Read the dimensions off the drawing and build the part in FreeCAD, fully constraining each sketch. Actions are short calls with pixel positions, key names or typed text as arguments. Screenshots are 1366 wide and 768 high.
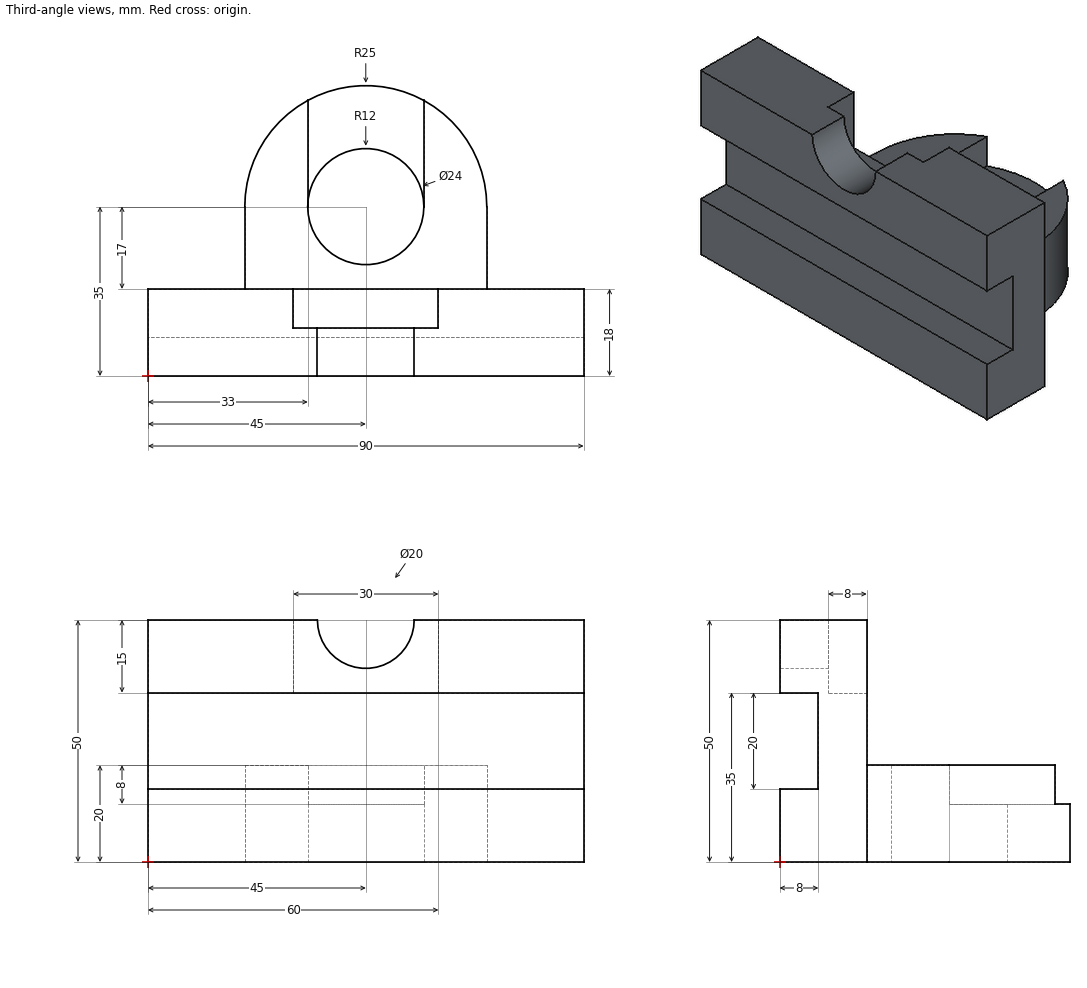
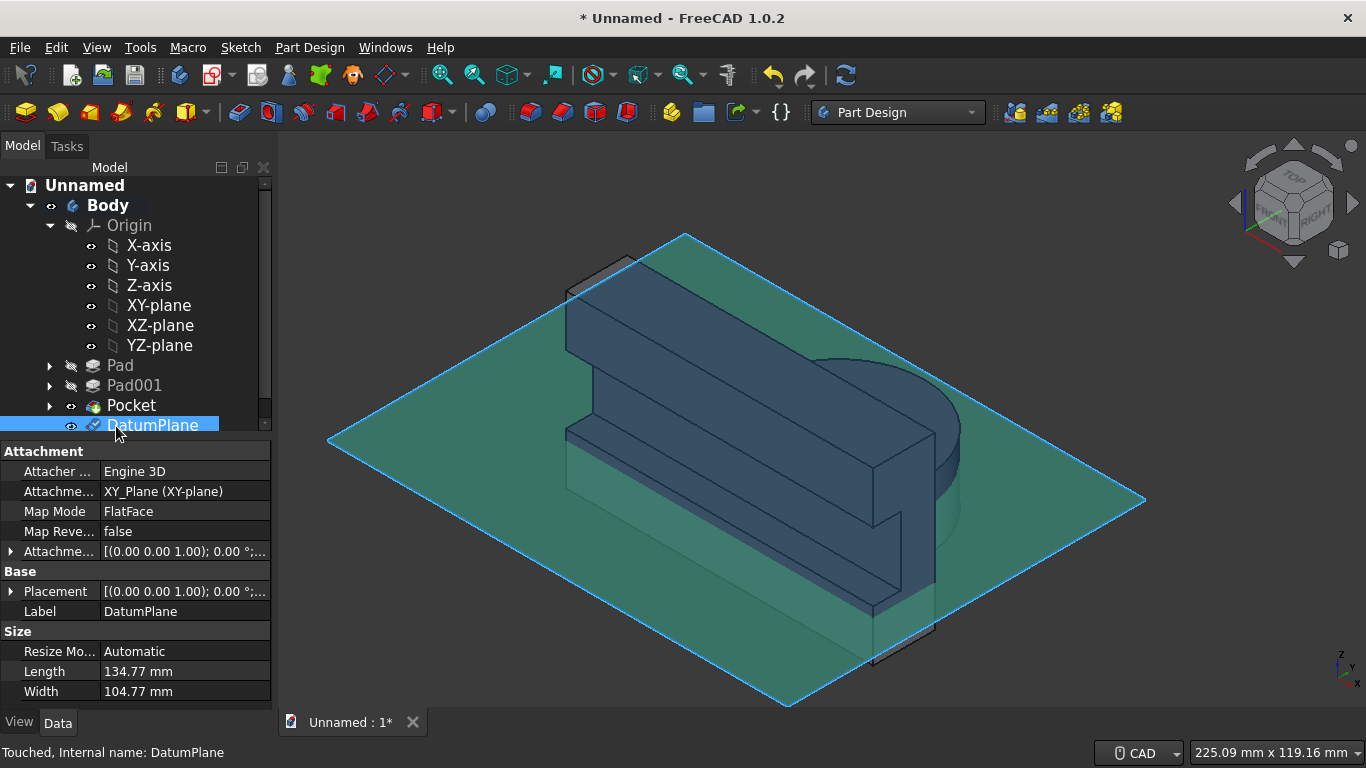
click(212, 76)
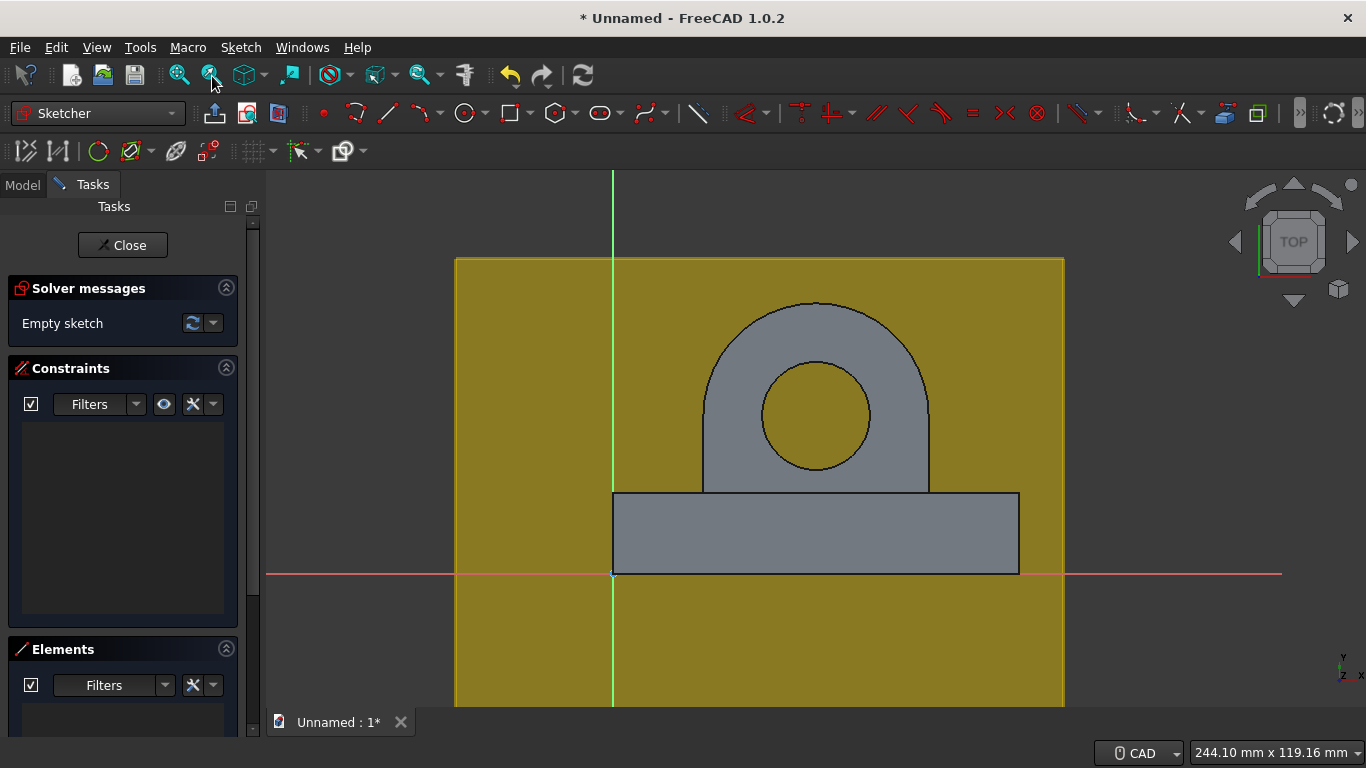
key(q)
key(s)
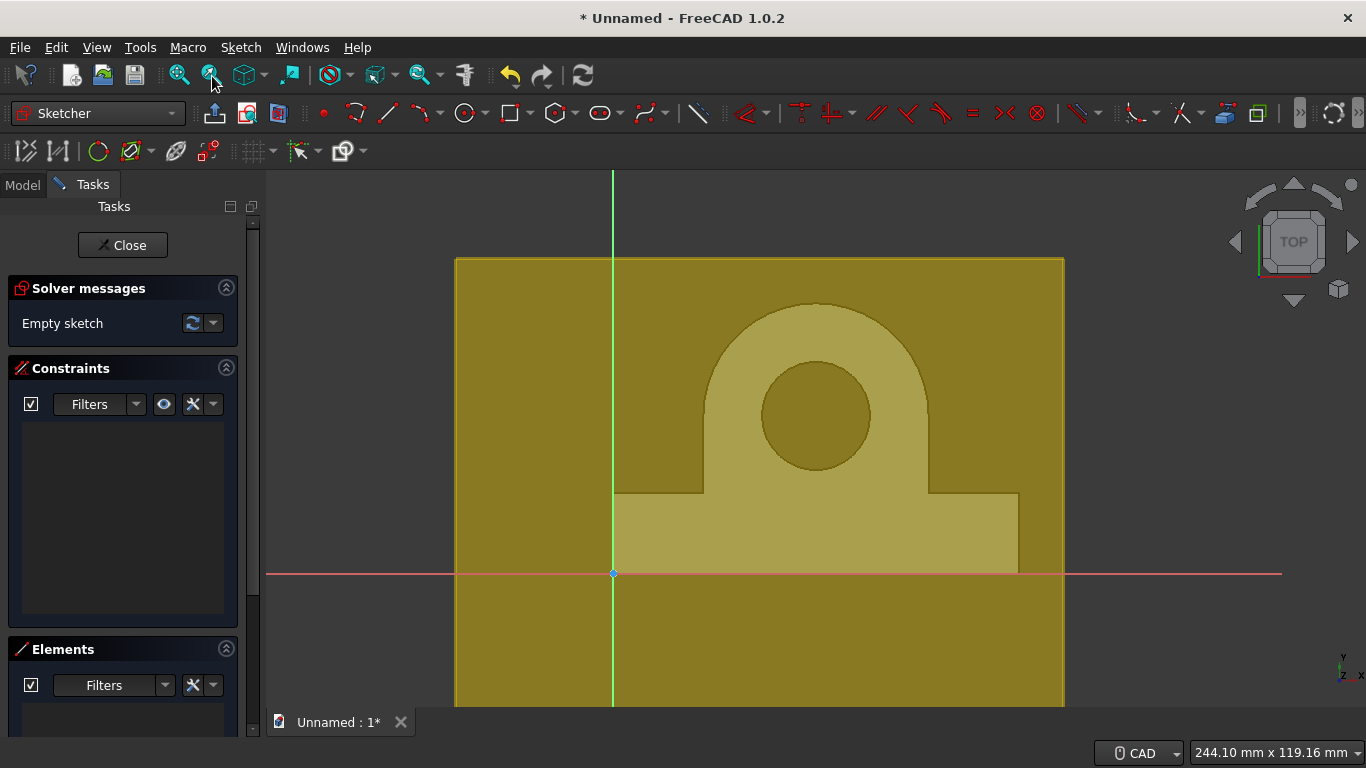
click(388, 114)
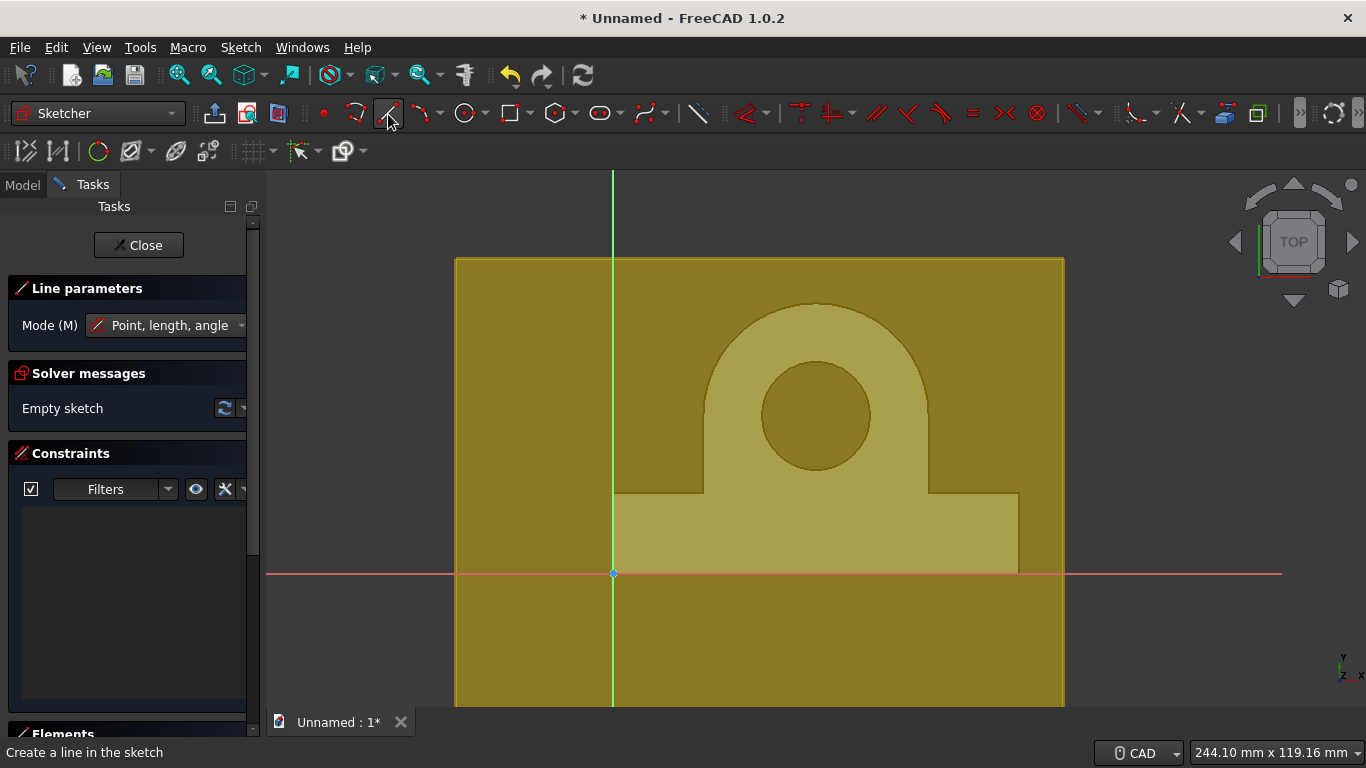
click(762, 317)
click(762, 416)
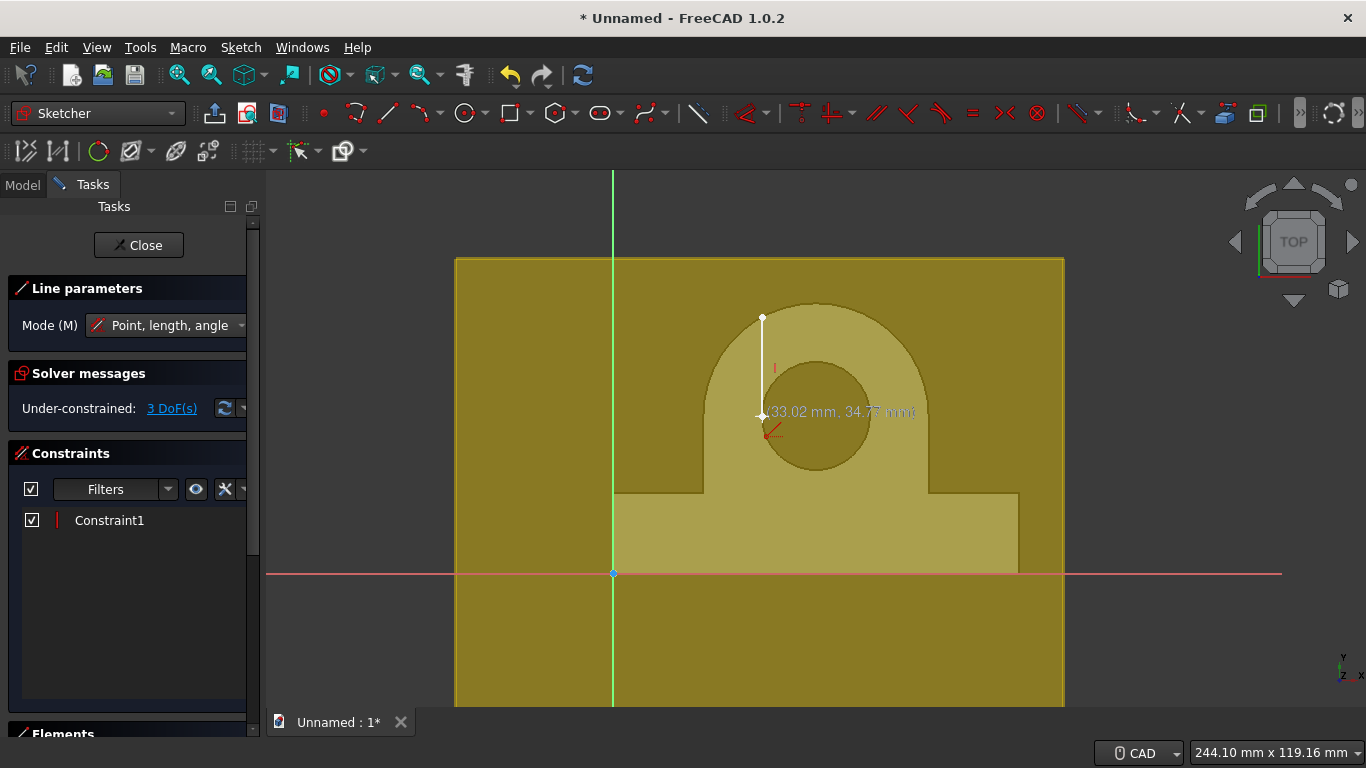
click(870, 416)
click(870, 317)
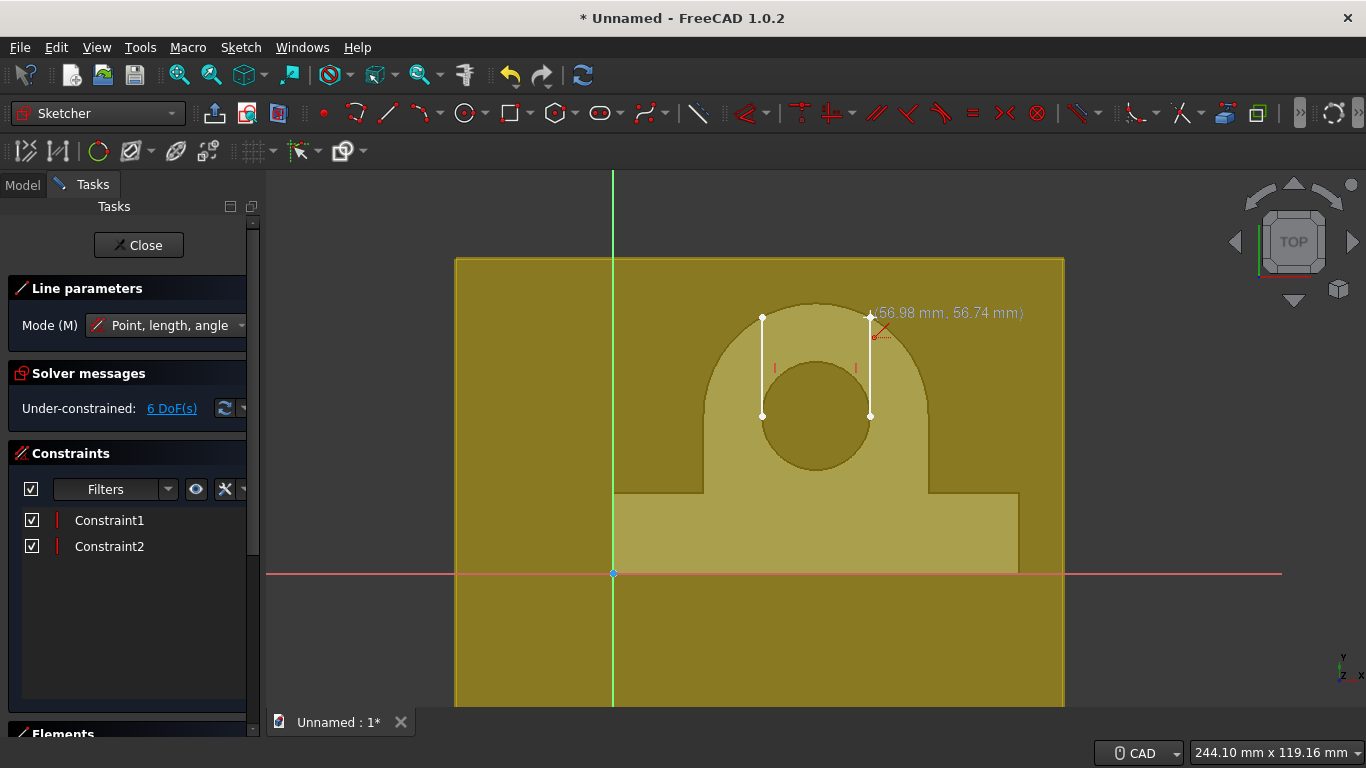
key(g)
key(3)
key(a)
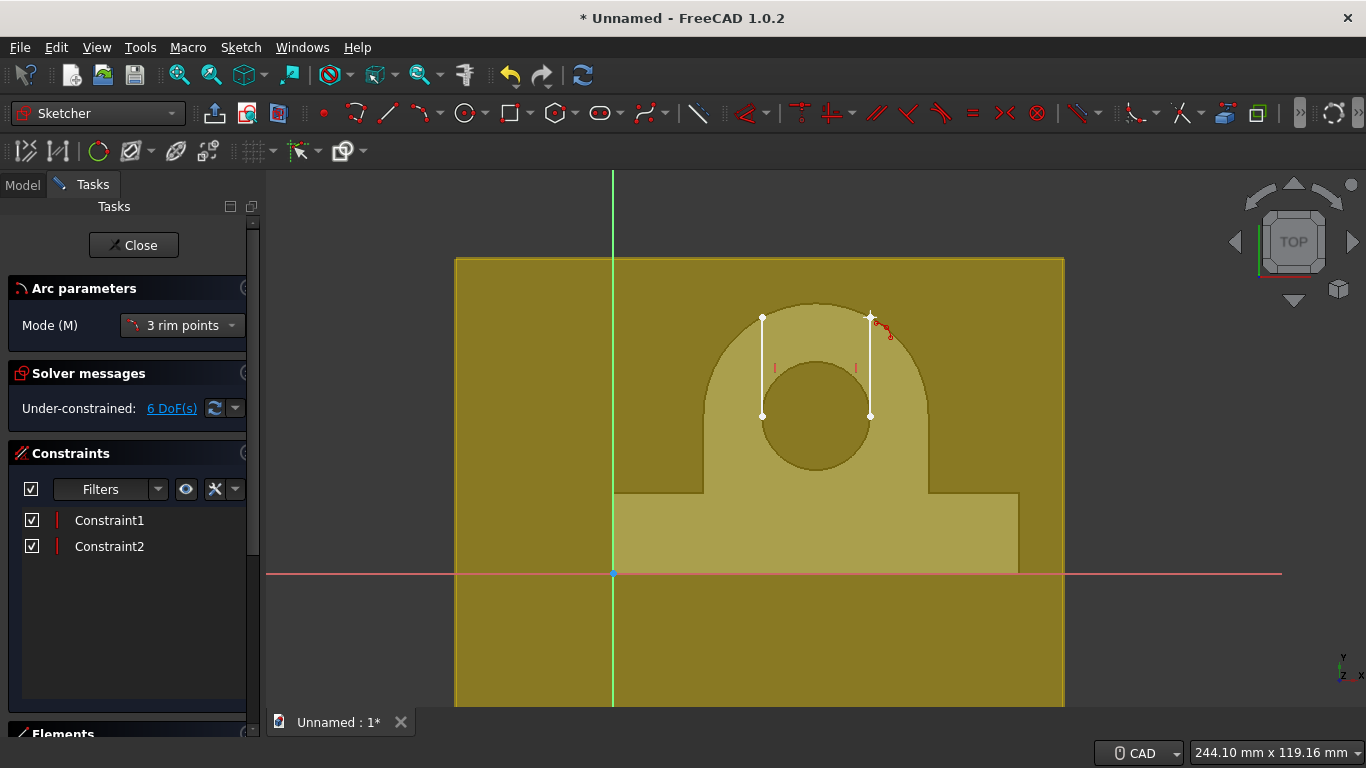
click(762, 417)
click(870, 417)
click(816, 362)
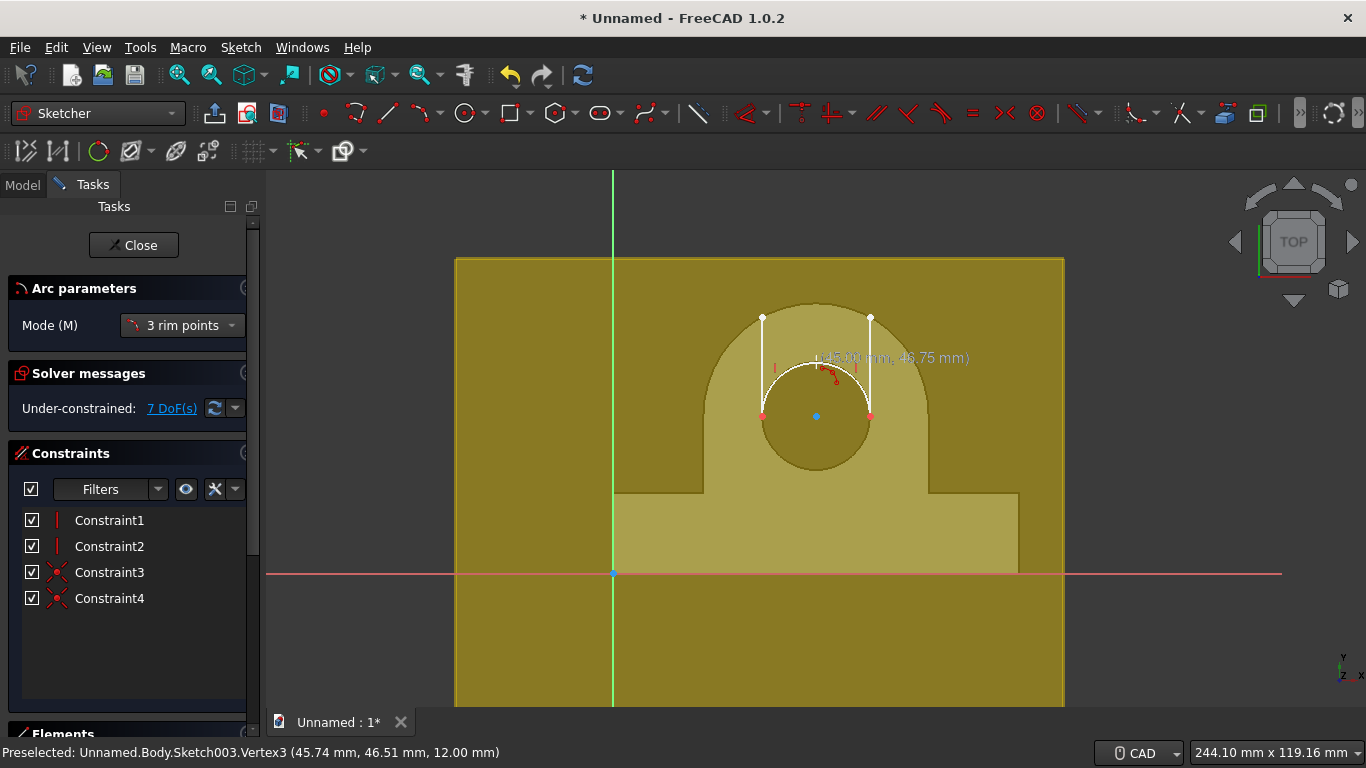
click(870, 318)
click(762, 318)
click(816, 303)
key(Escape)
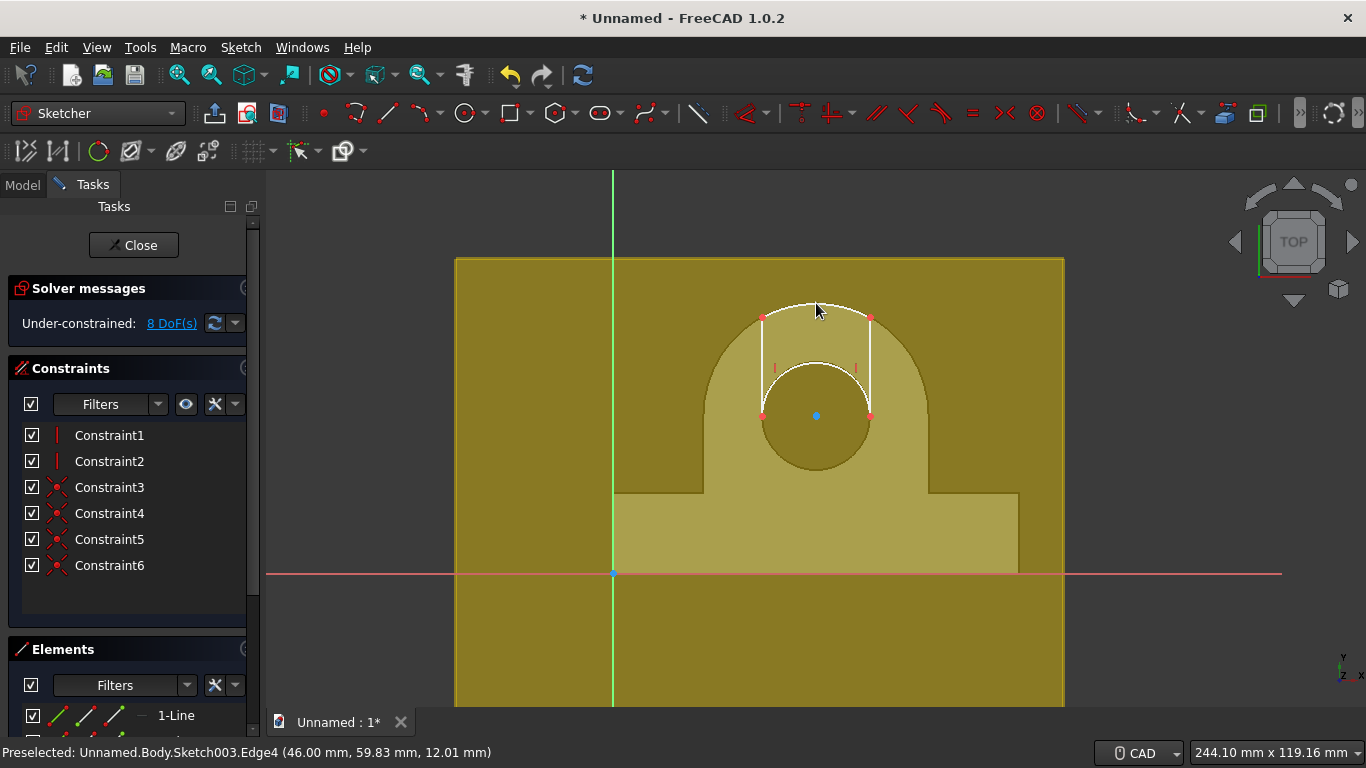
click(762, 348)